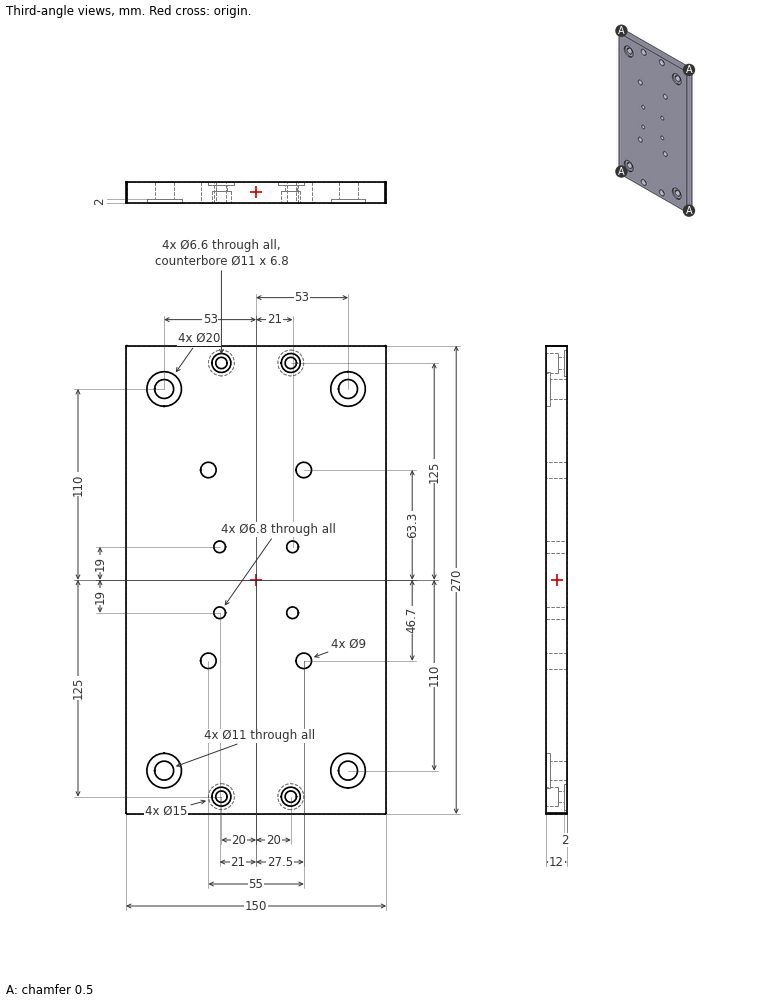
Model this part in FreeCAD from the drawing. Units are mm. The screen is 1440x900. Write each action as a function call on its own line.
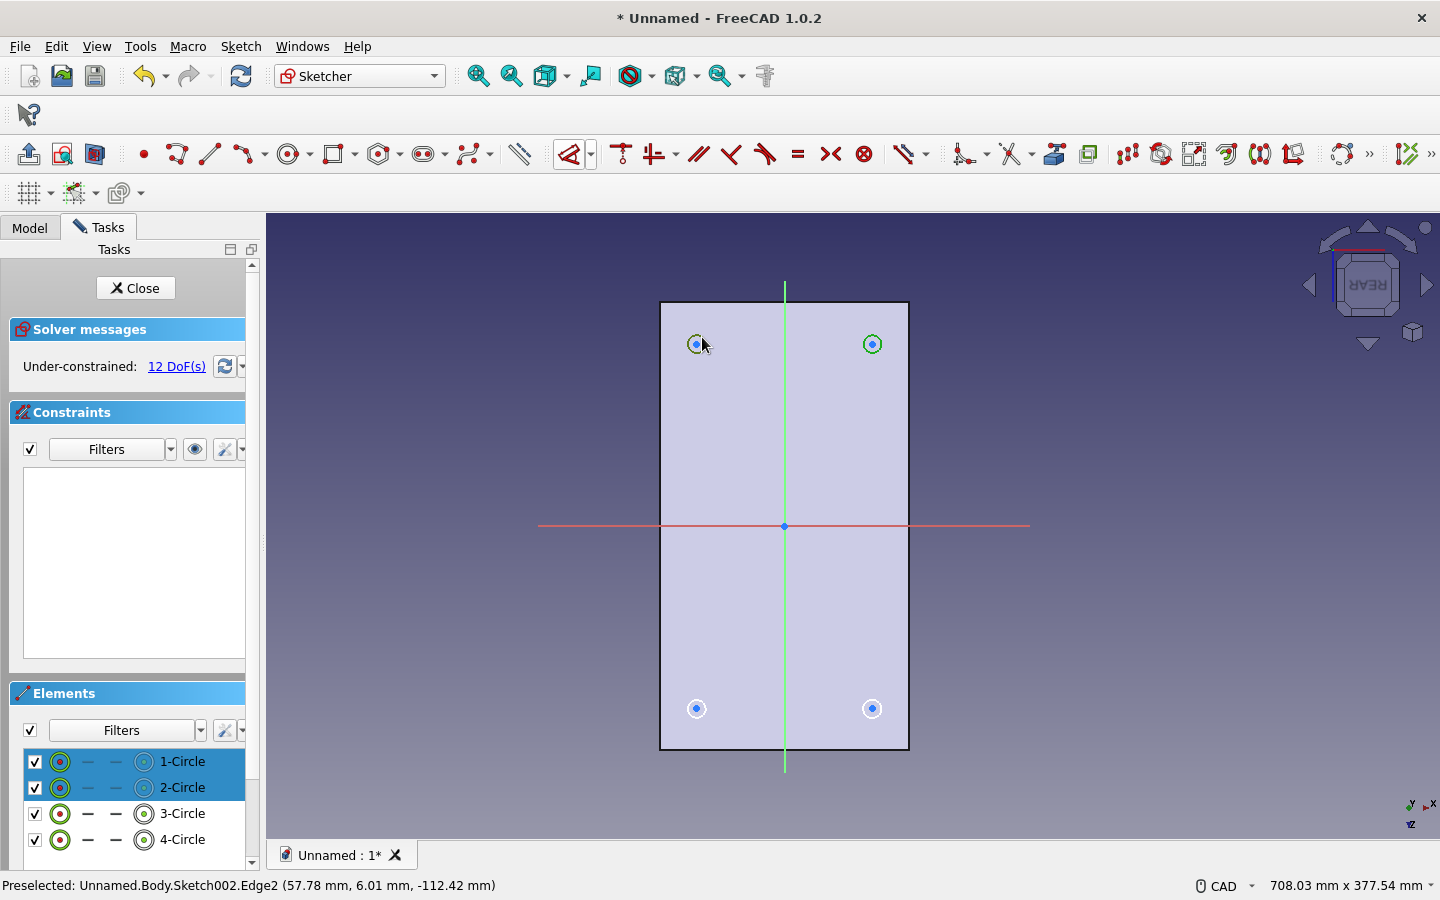
scroll(703, 703, up, 3)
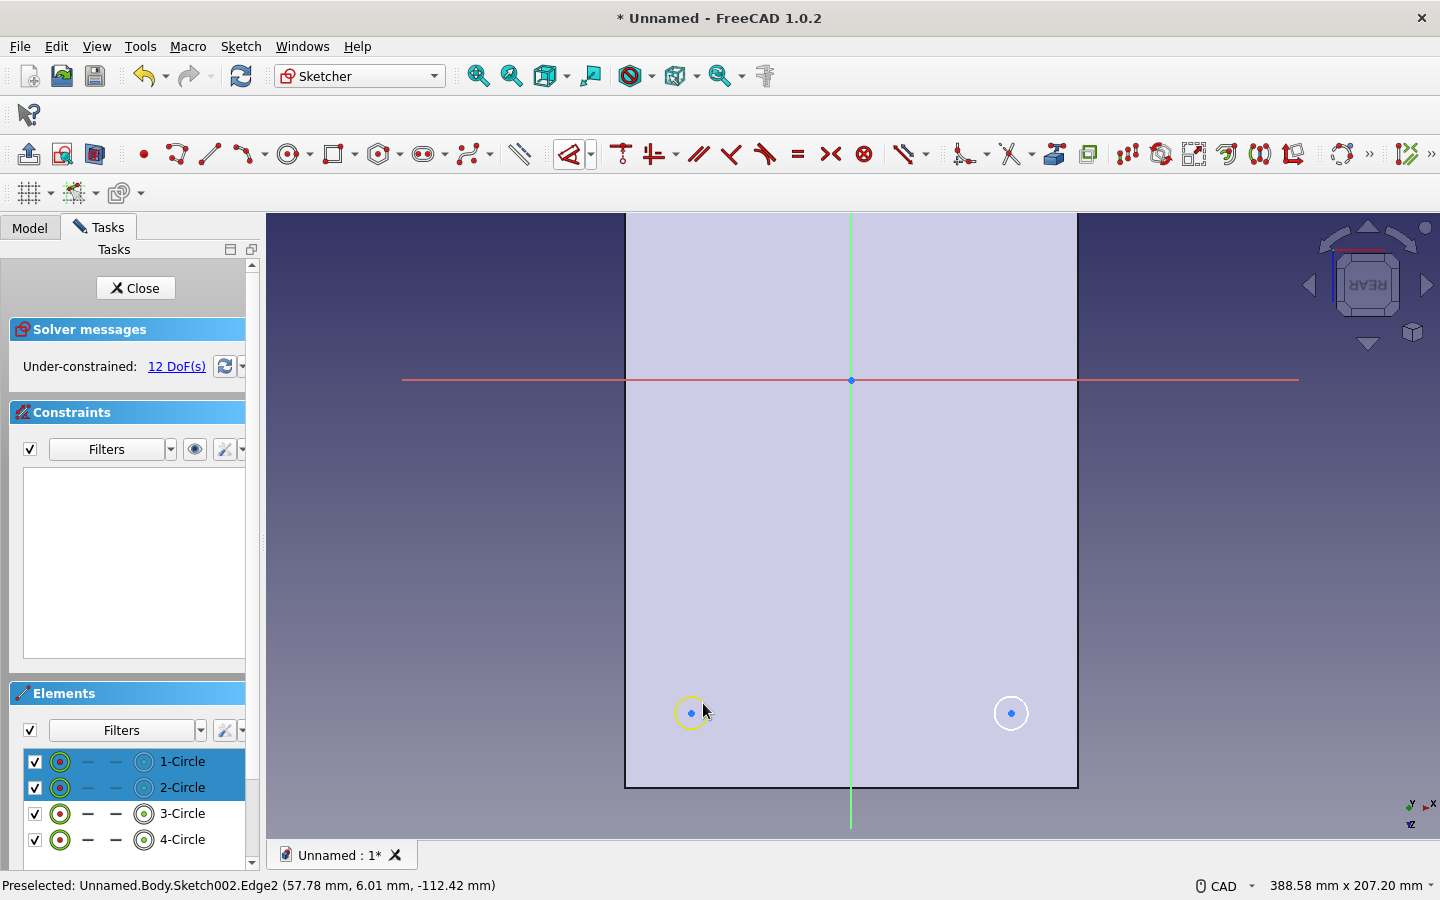
click(703, 702)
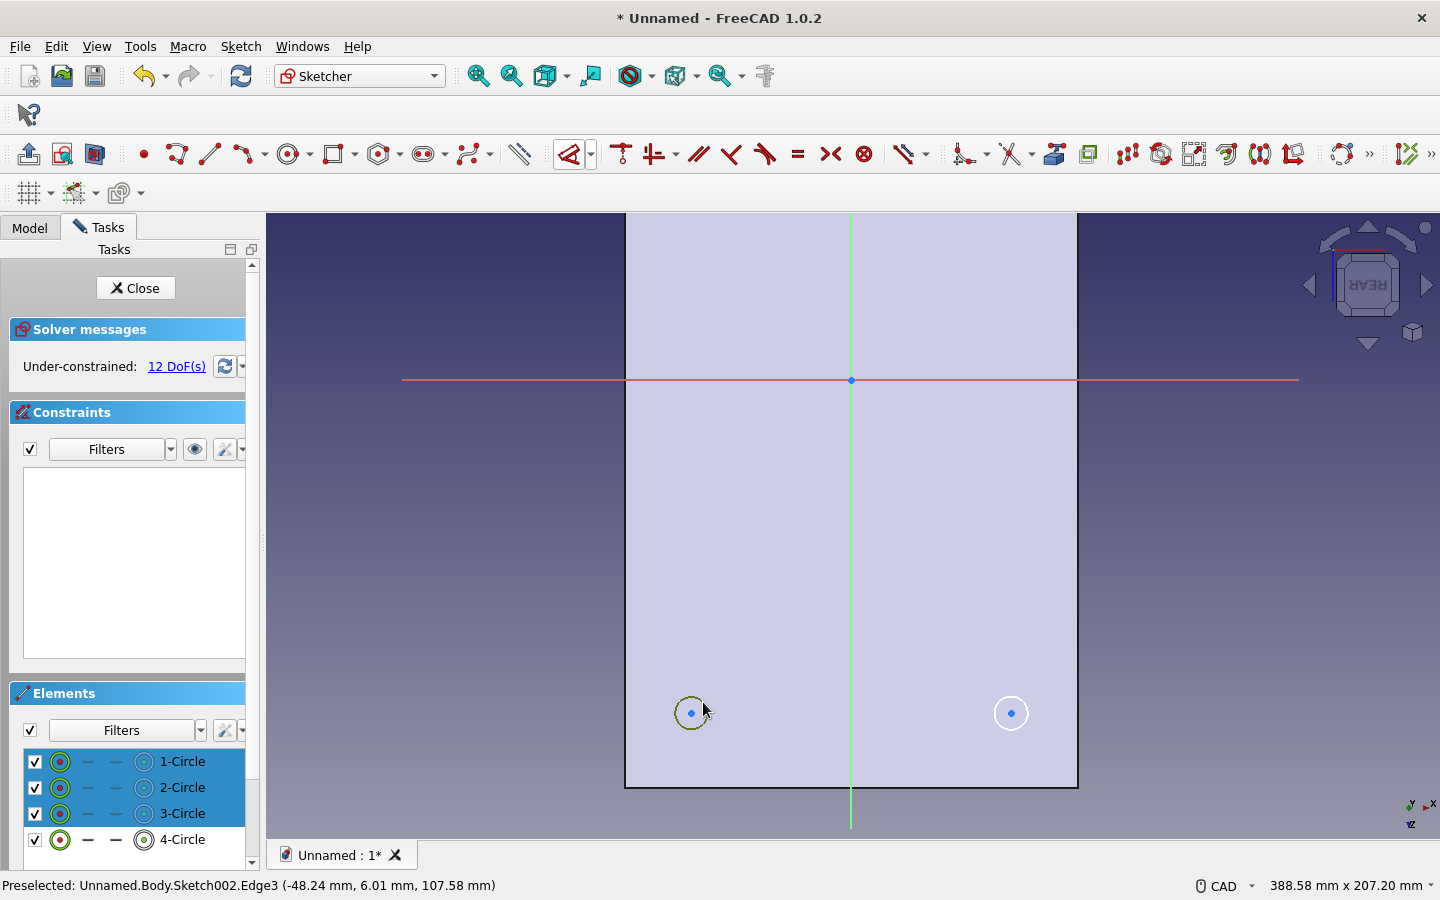
click(1023, 701)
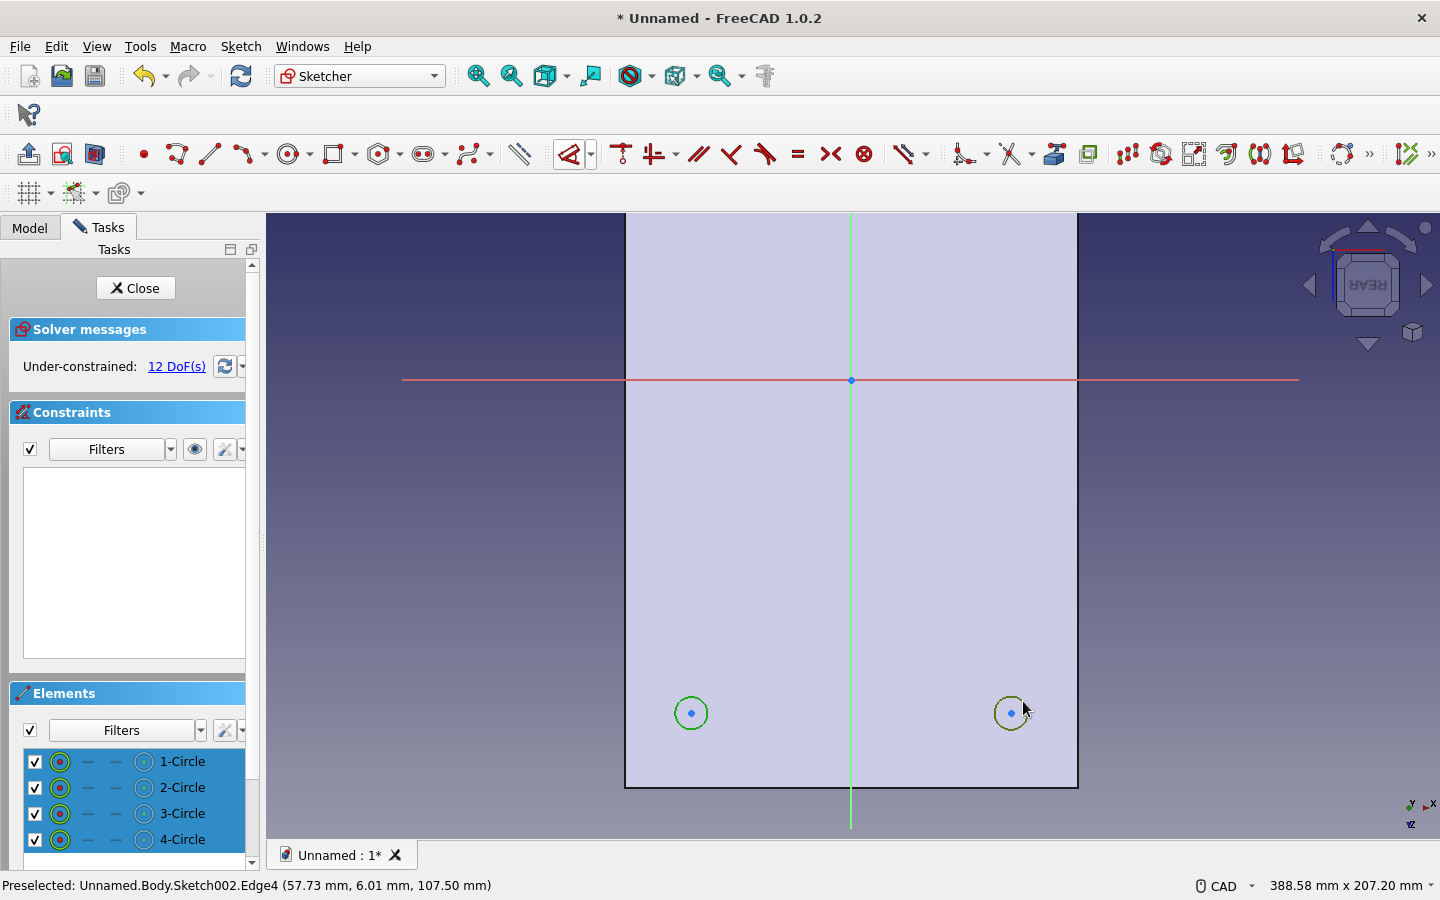
click(798, 154)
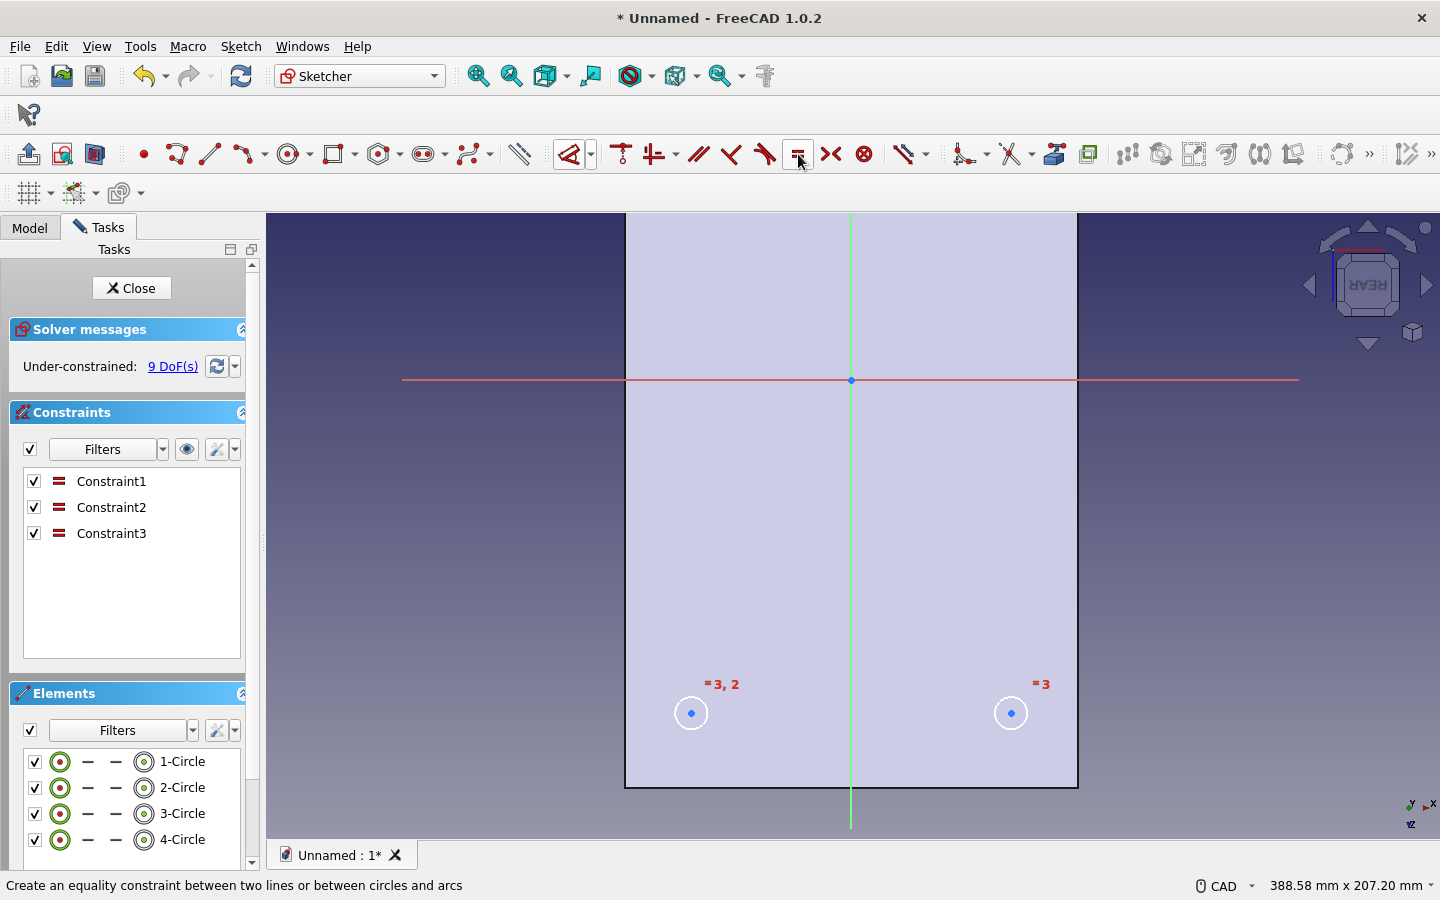
scroll(703, 703, down, 3)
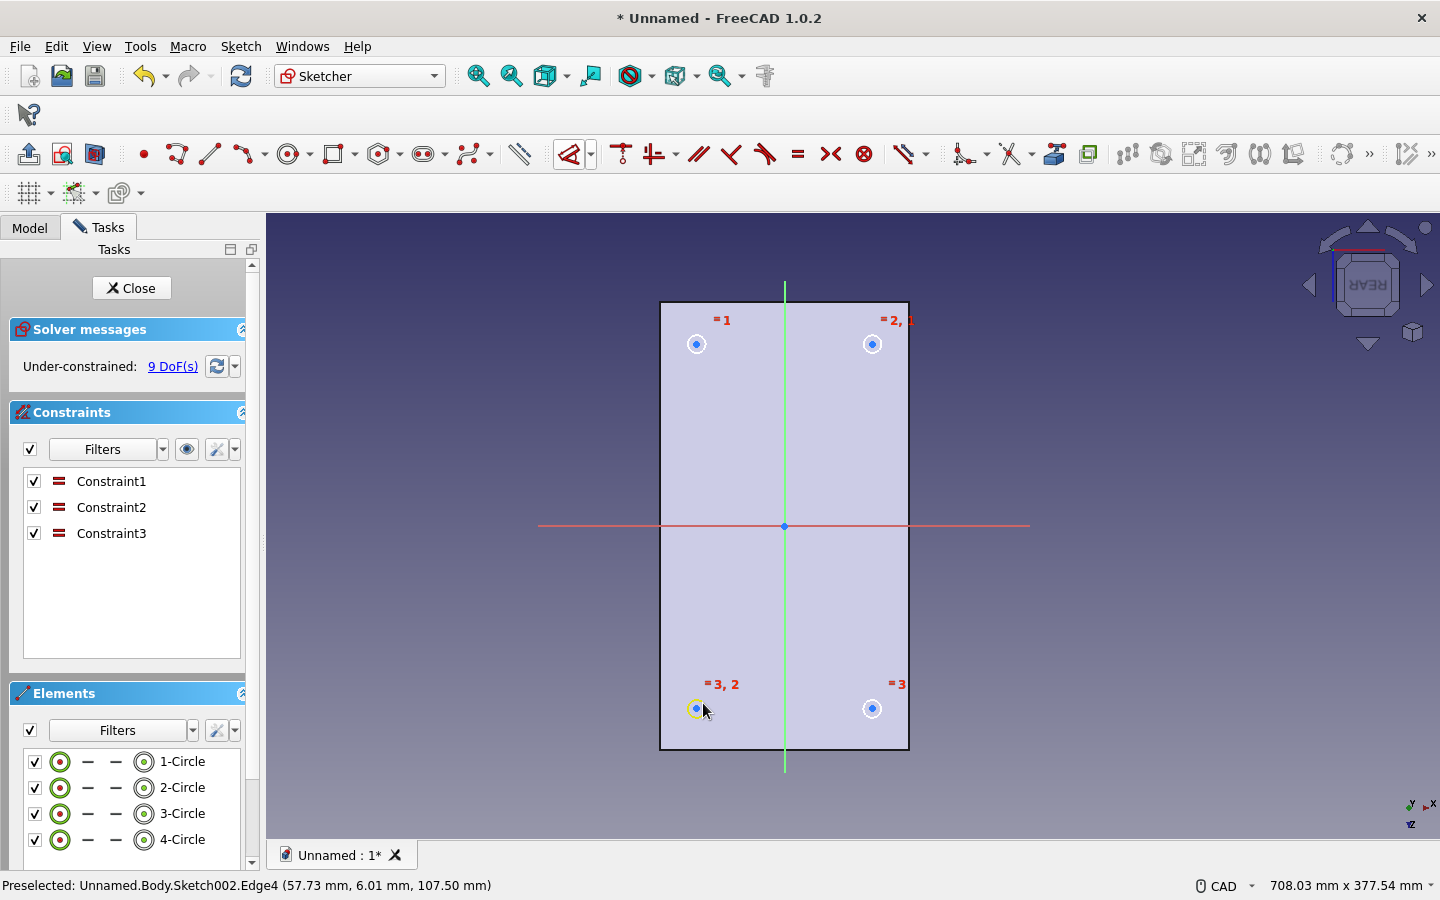
click(697, 344)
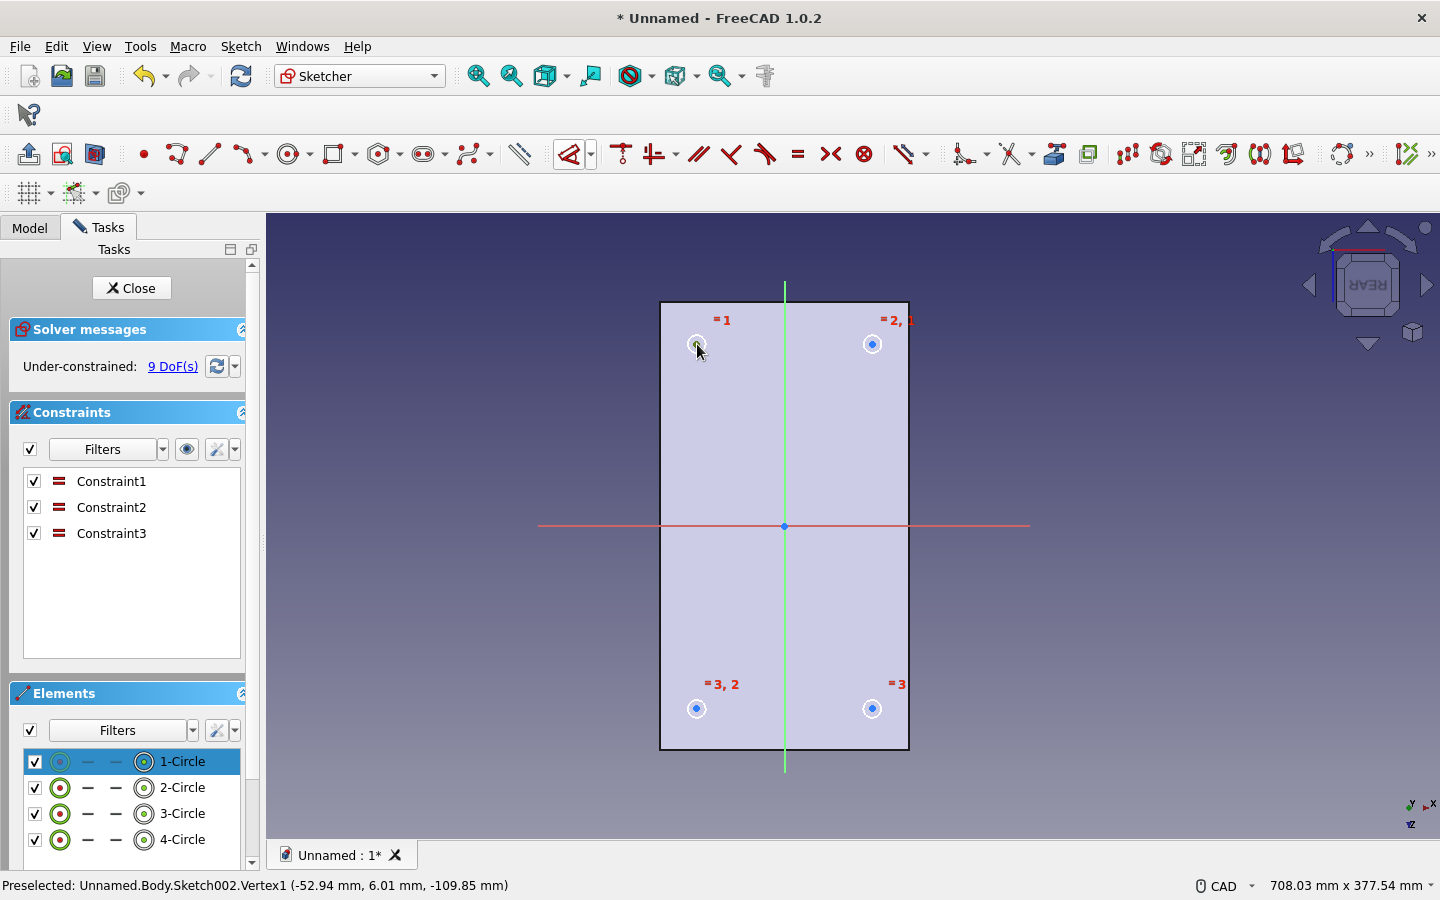
click(873, 344)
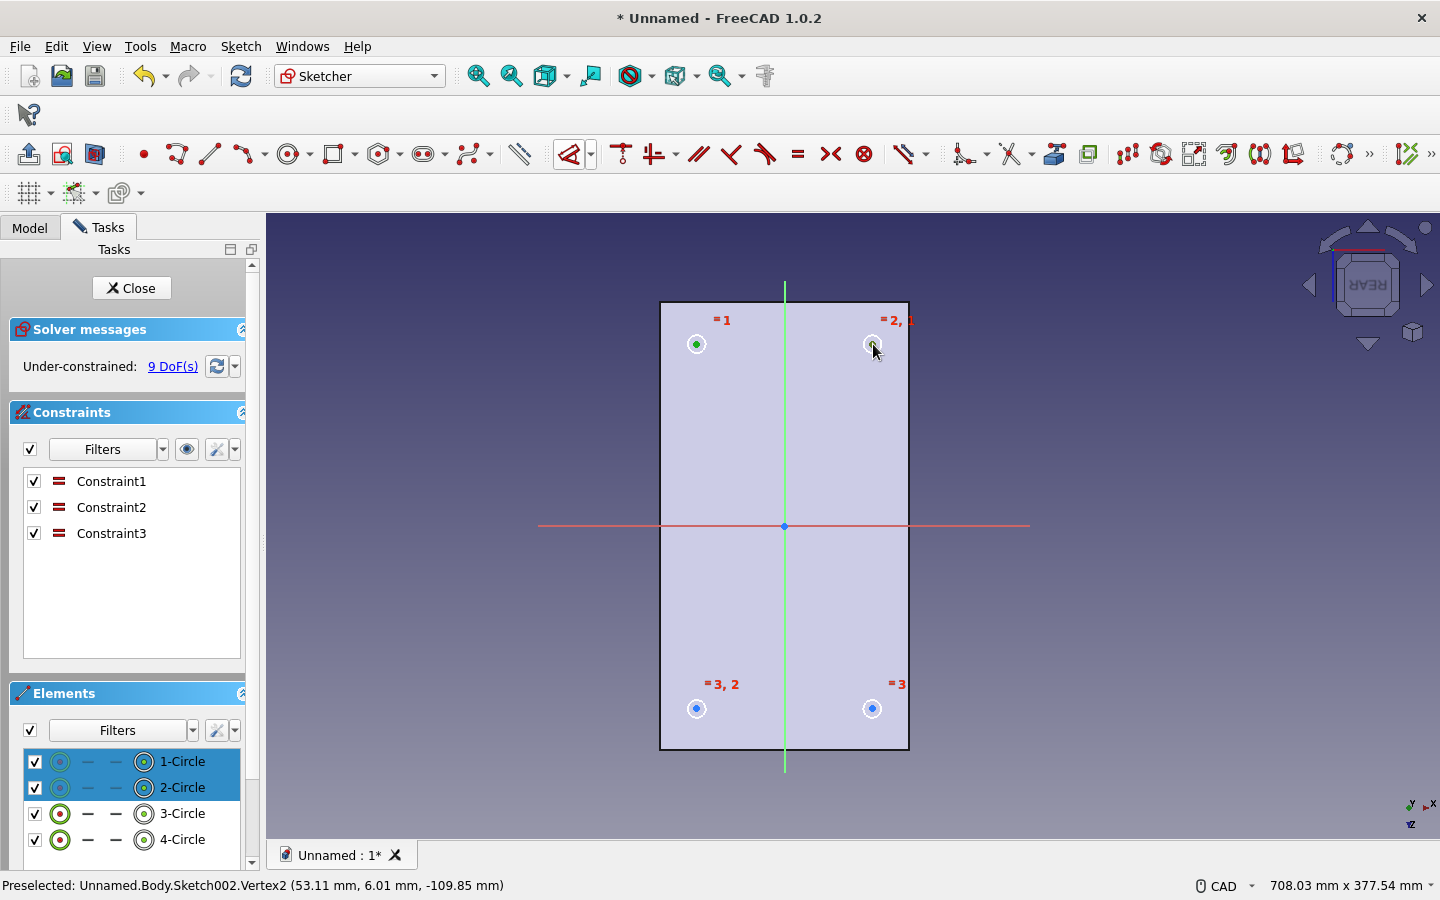
key(h)